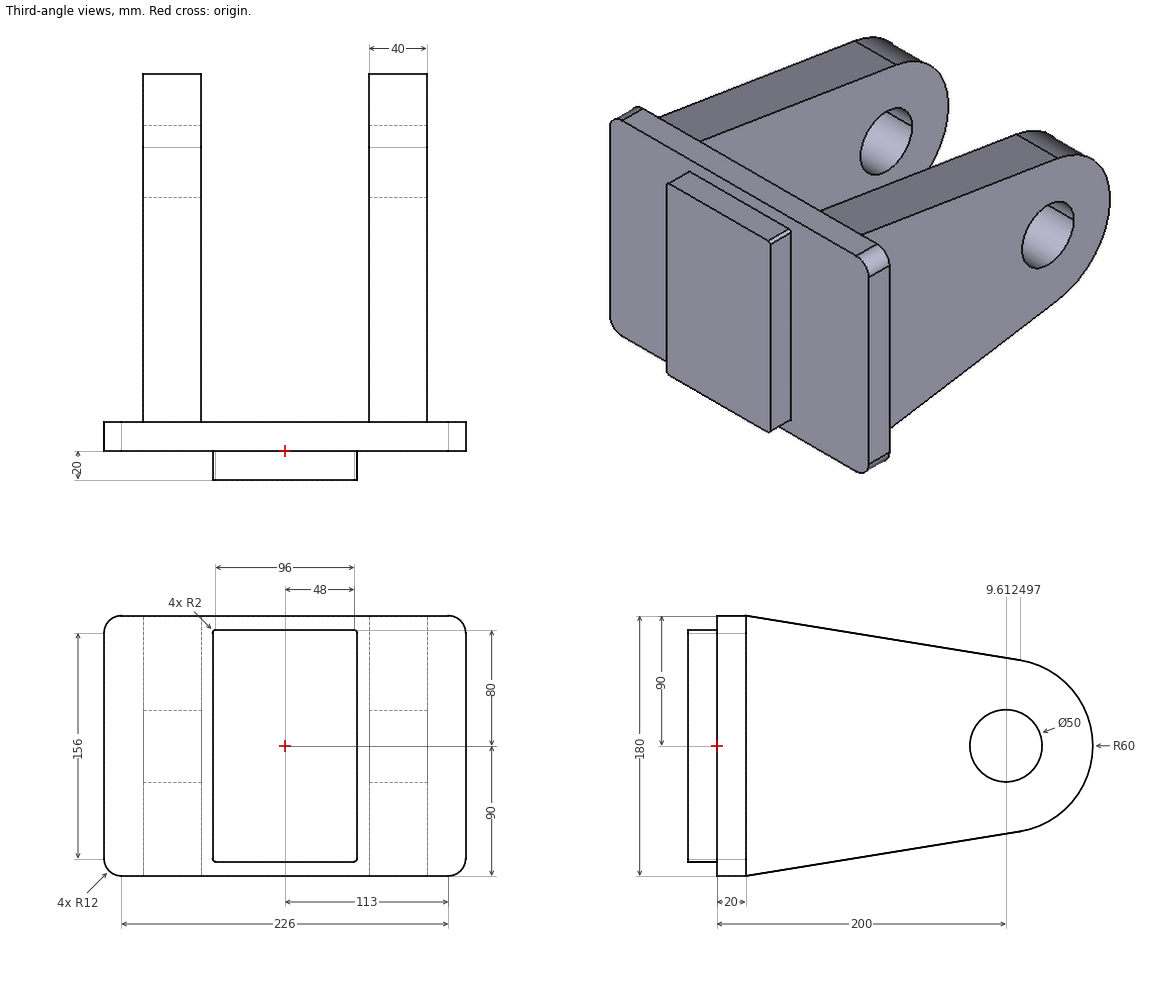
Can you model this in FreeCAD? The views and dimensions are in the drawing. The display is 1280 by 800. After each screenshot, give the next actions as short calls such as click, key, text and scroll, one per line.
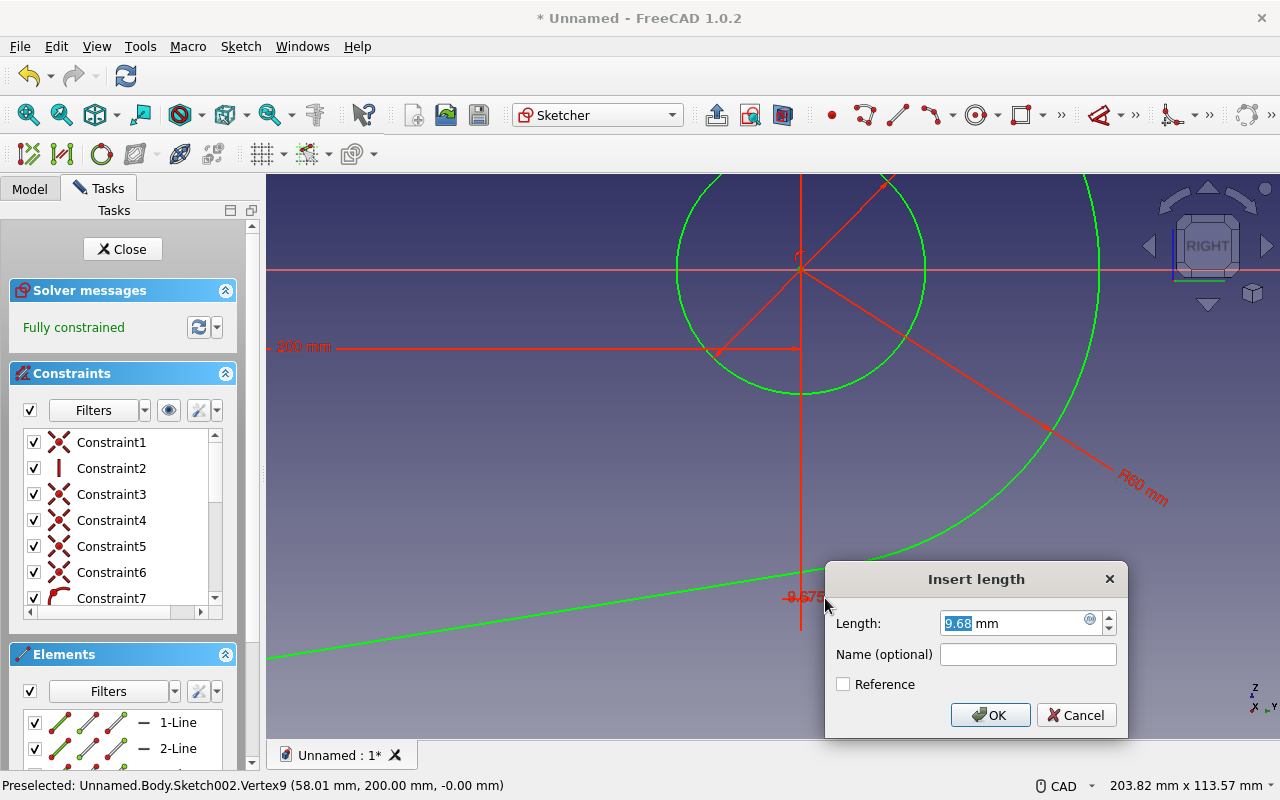
text(9.612497)
key(Return)
key(Escape)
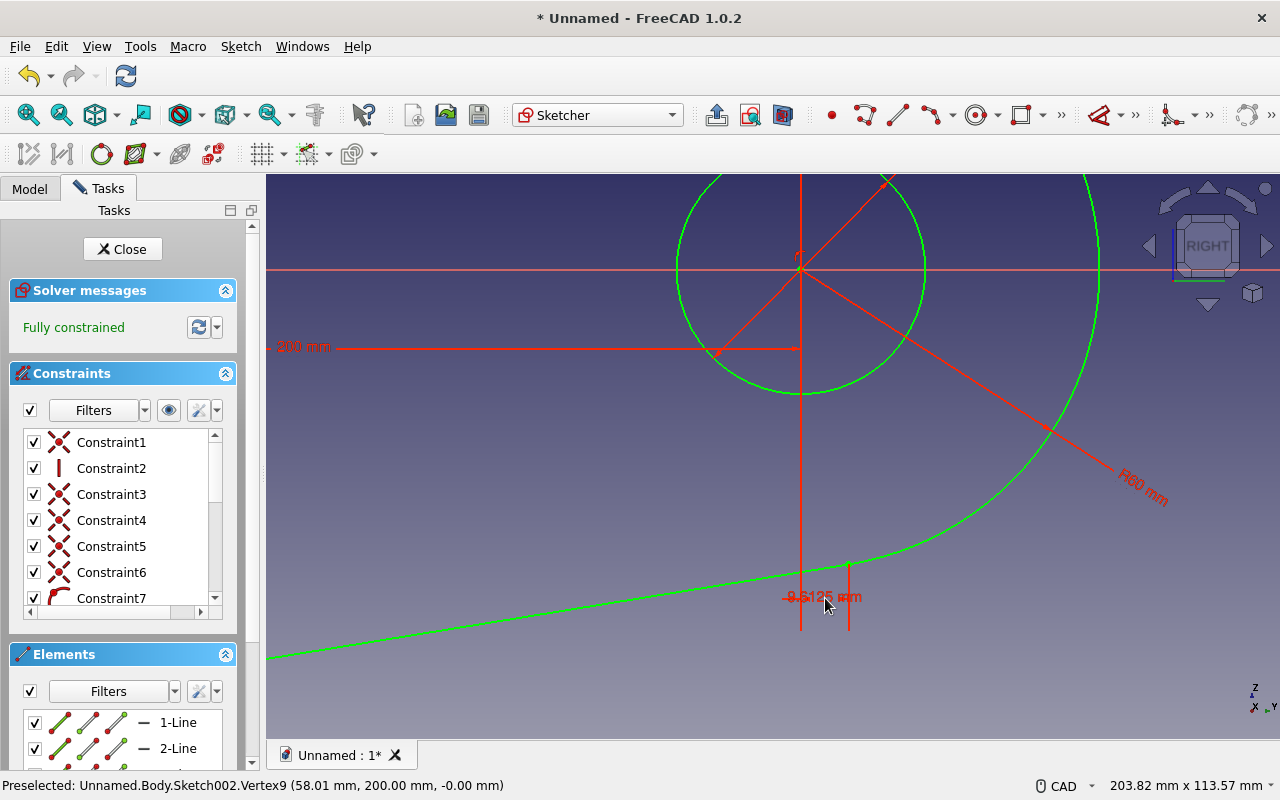
click(123, 249)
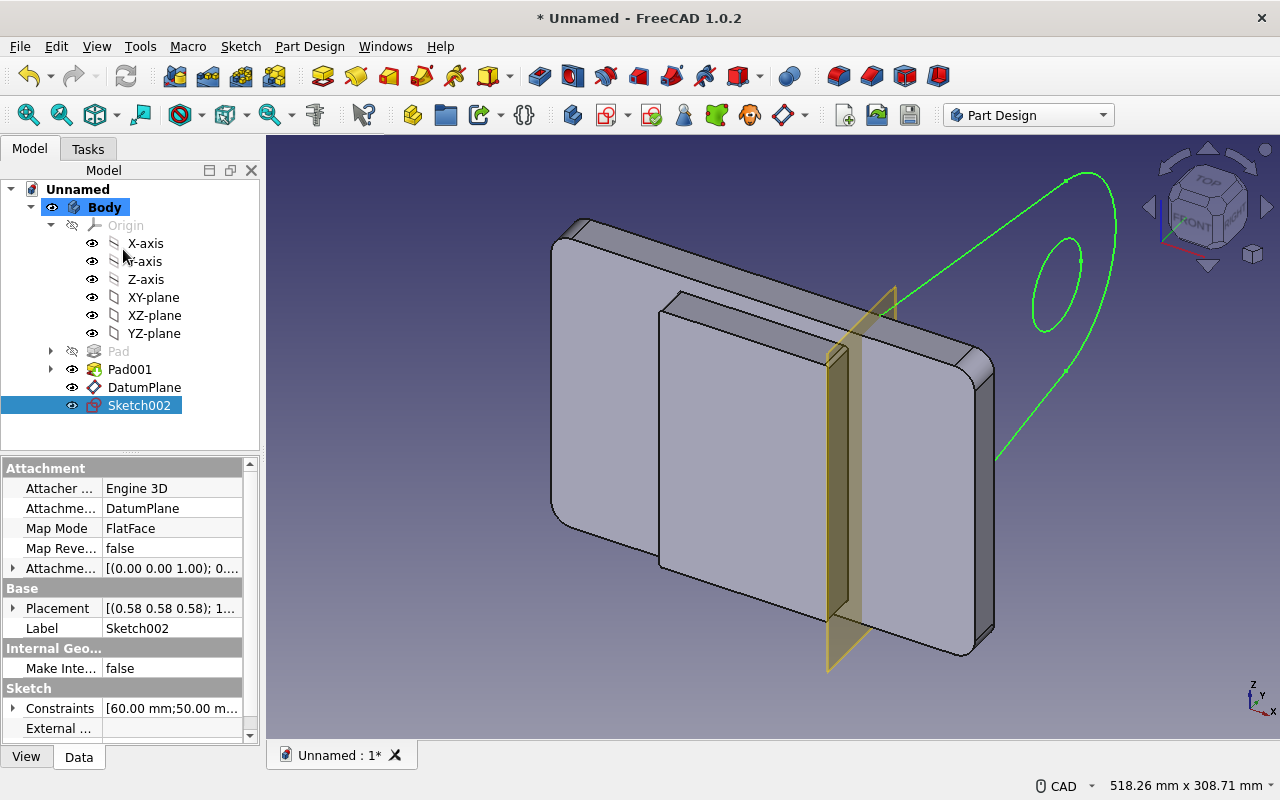
click(323, 76)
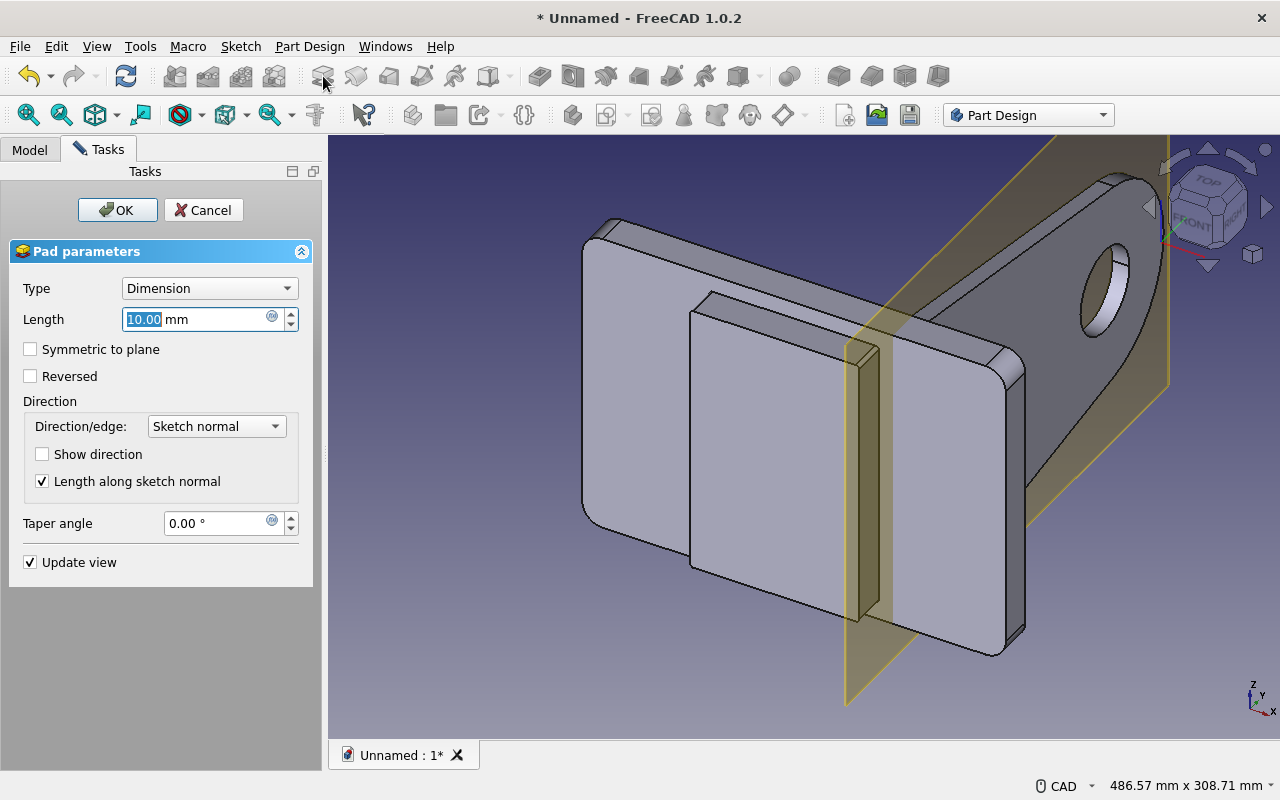
text(40)
key(Tab)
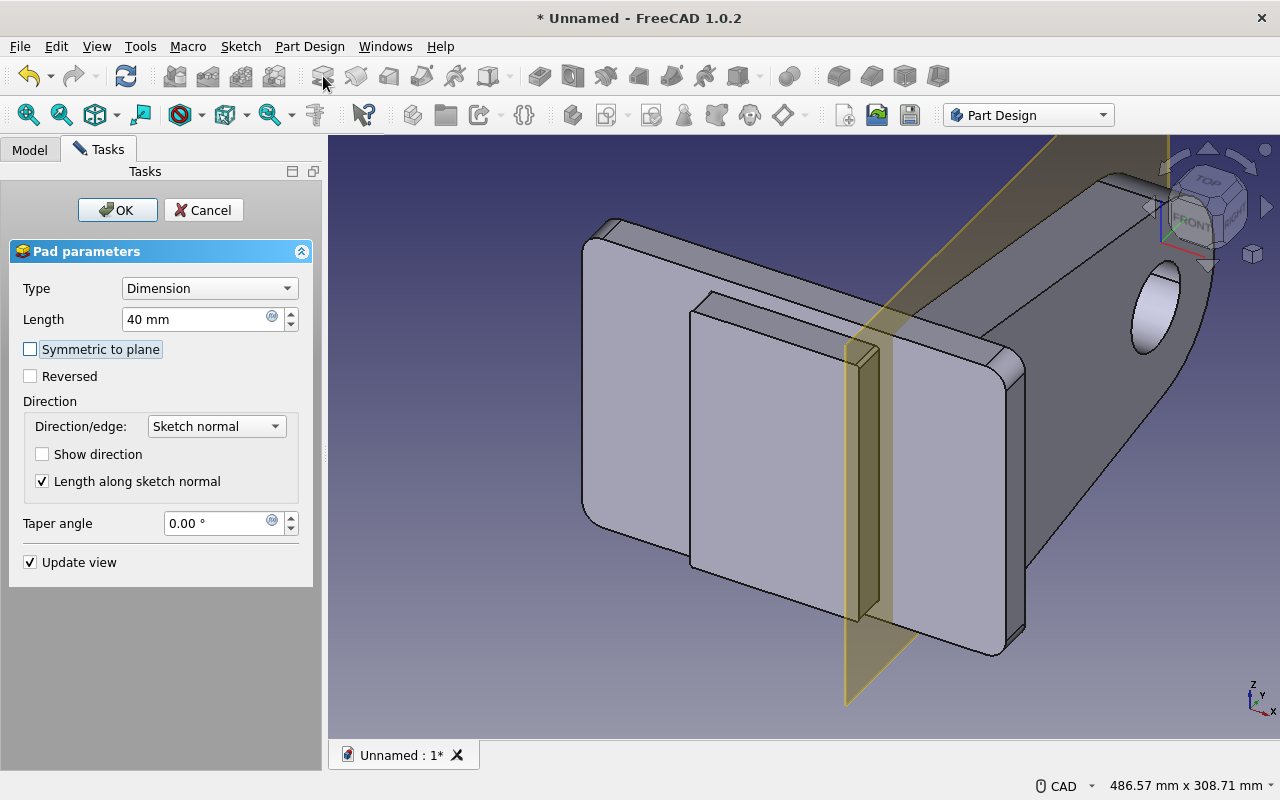
click(118, 210)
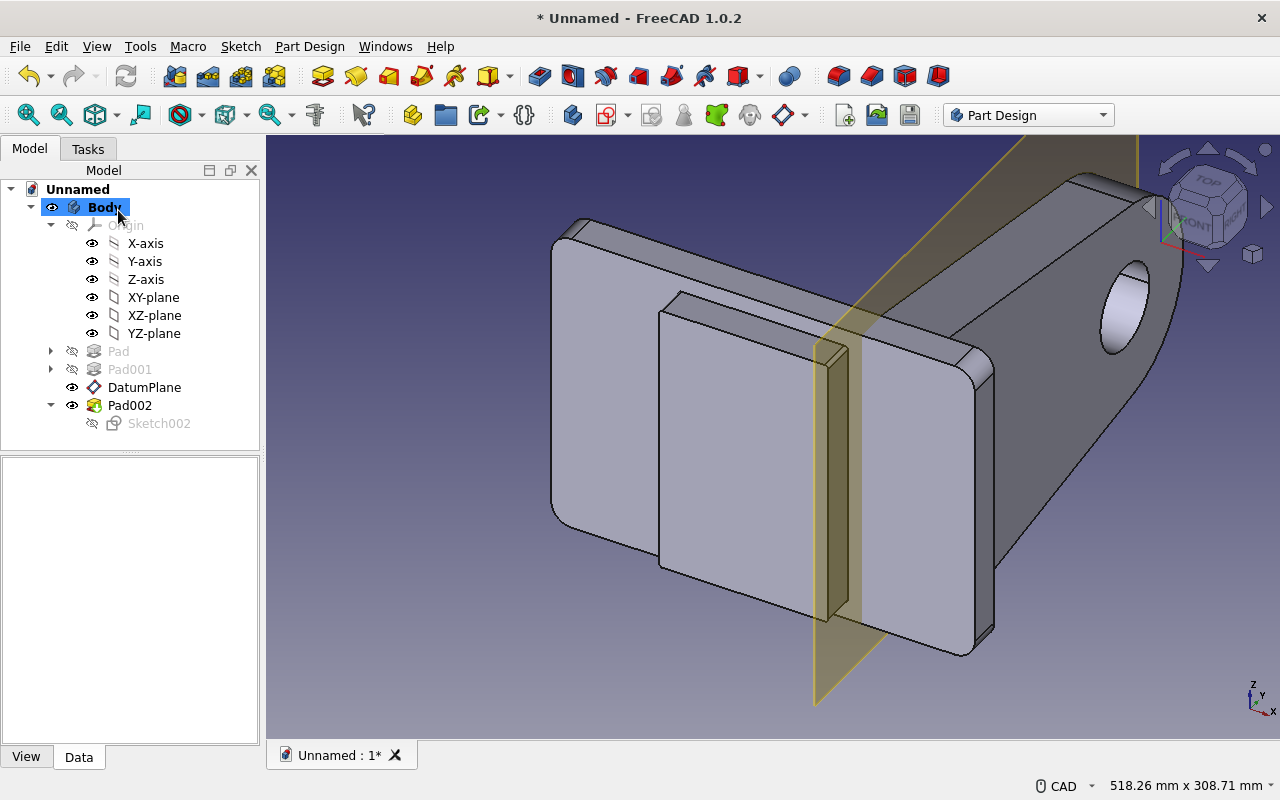
click(117, 387)
key(space)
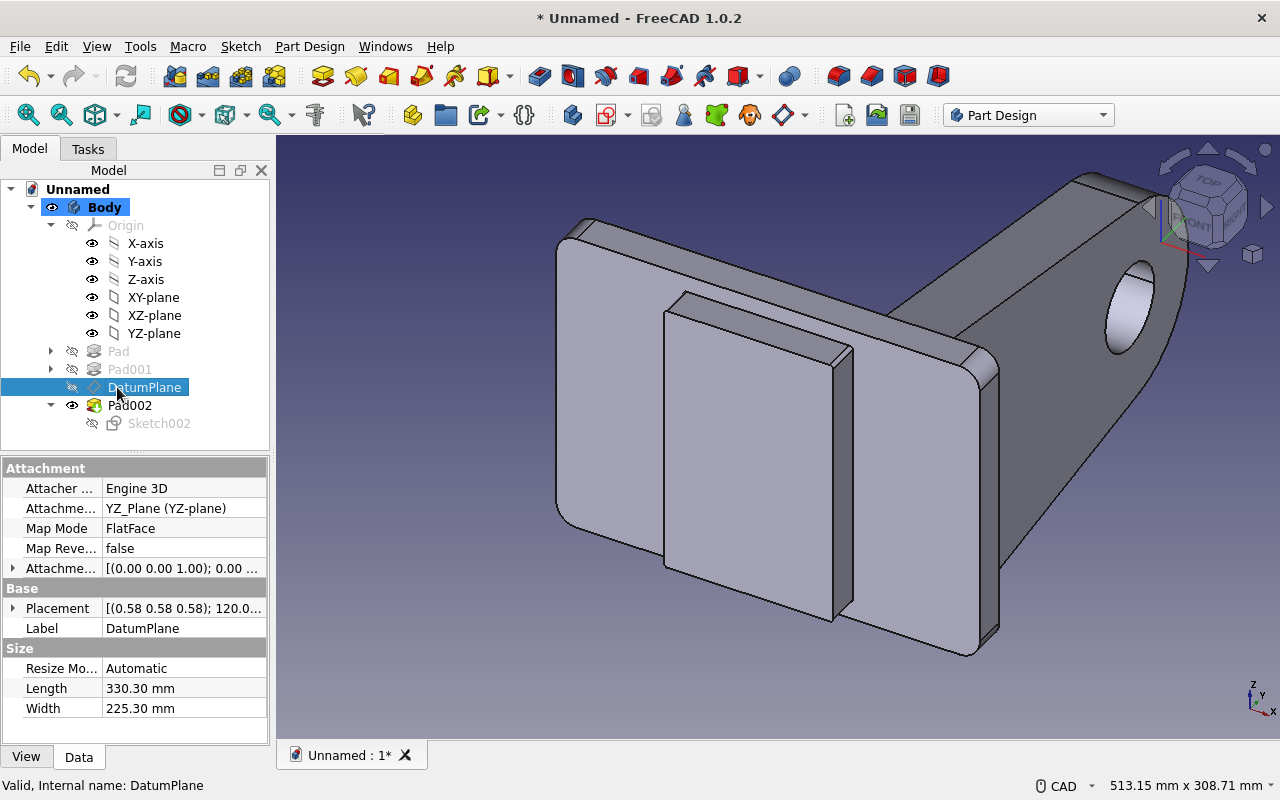
click(29, 116)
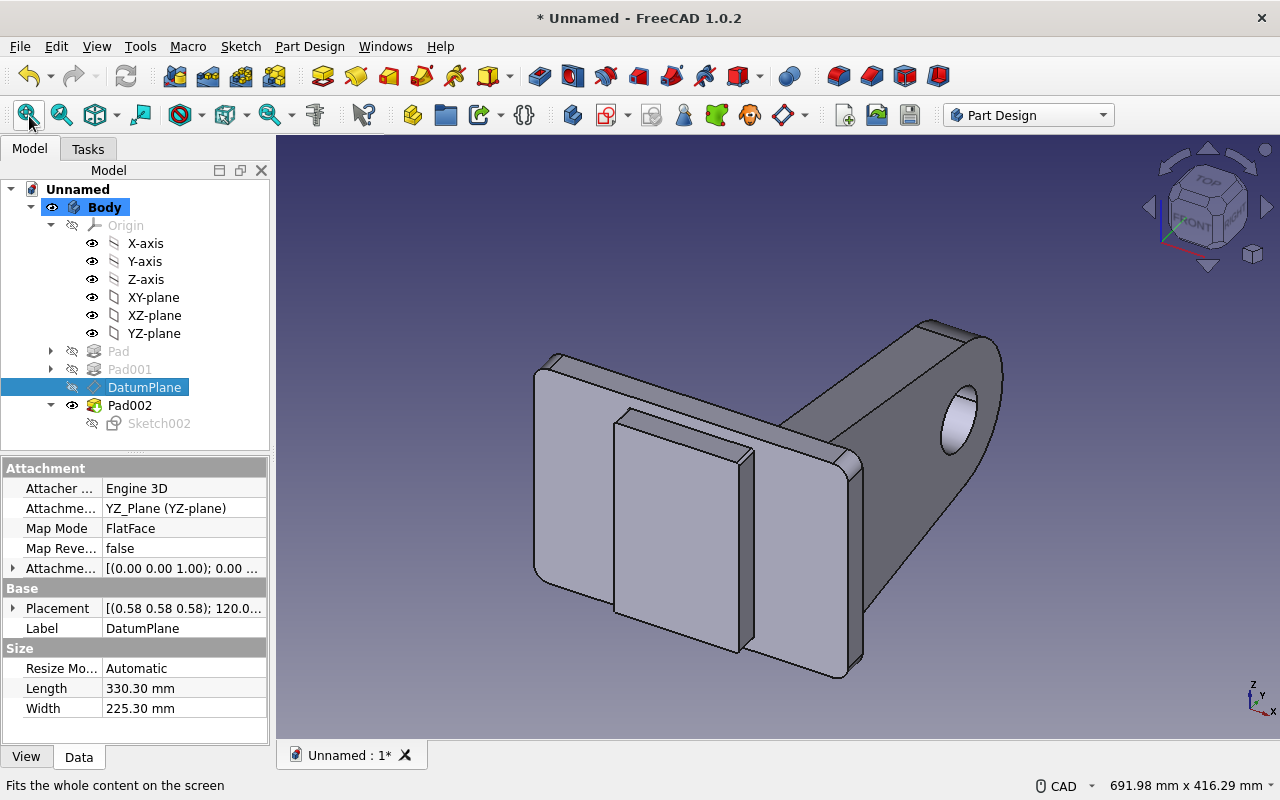
click(117, 405)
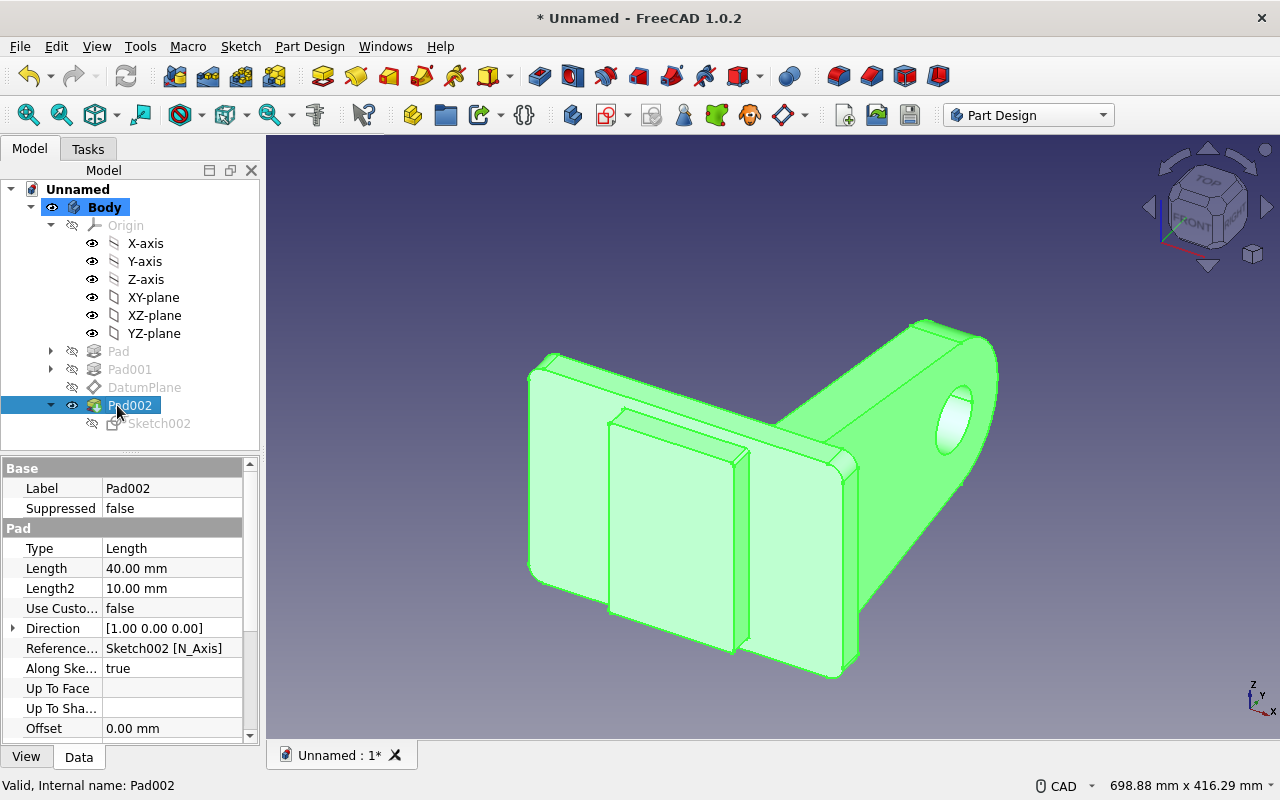
click(175, 76)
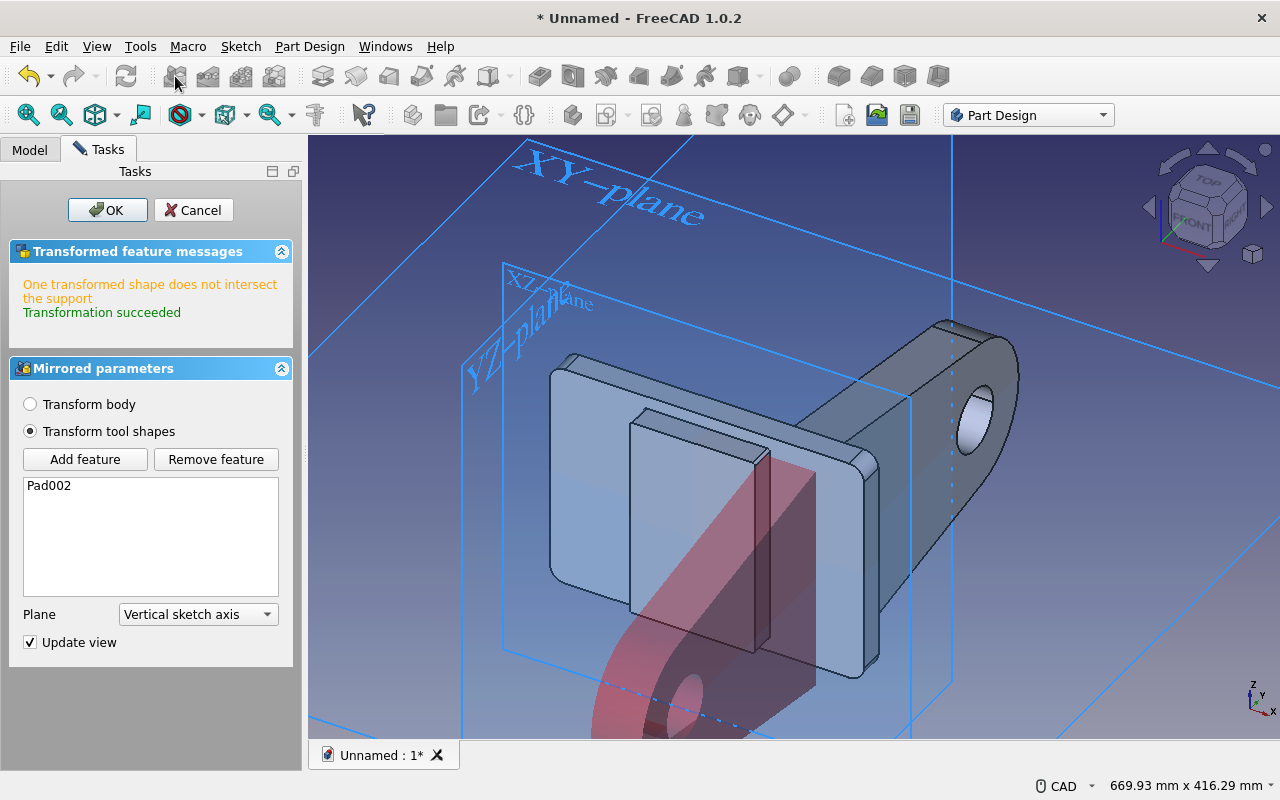
click(199, 614)